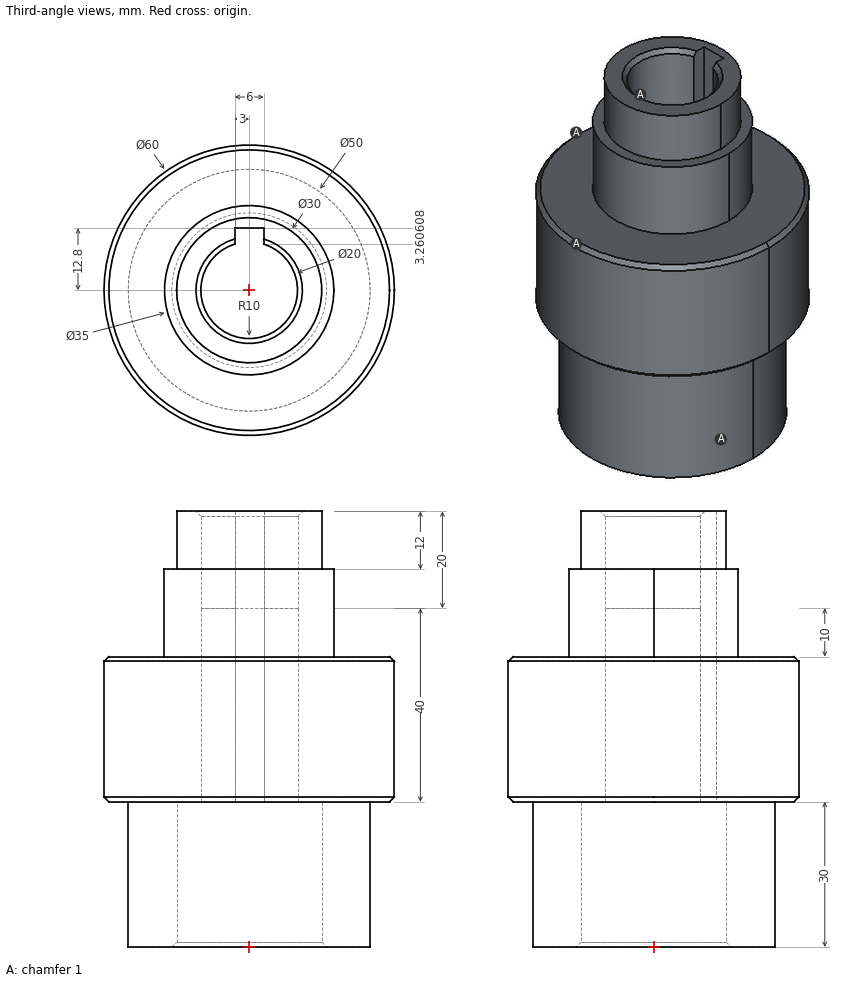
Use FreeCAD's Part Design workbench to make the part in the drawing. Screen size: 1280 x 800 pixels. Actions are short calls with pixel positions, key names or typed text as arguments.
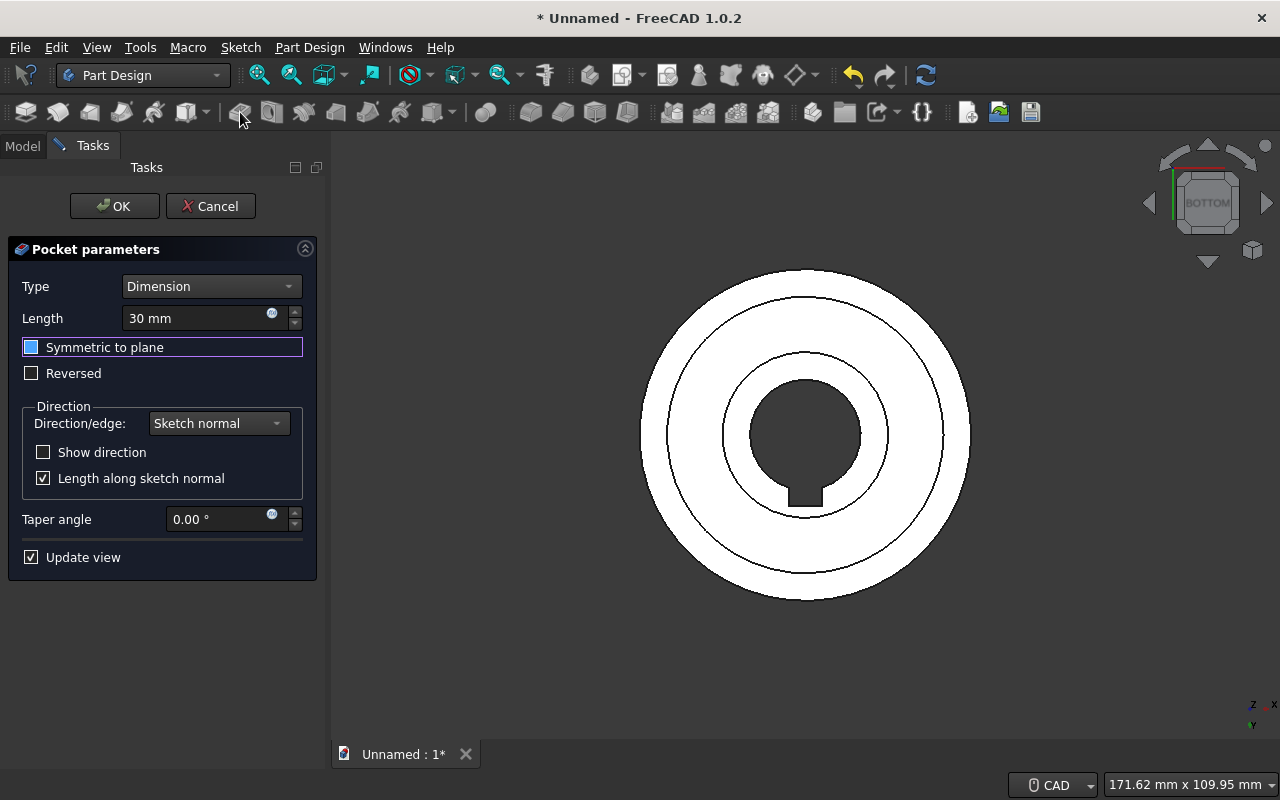
click(115, 206)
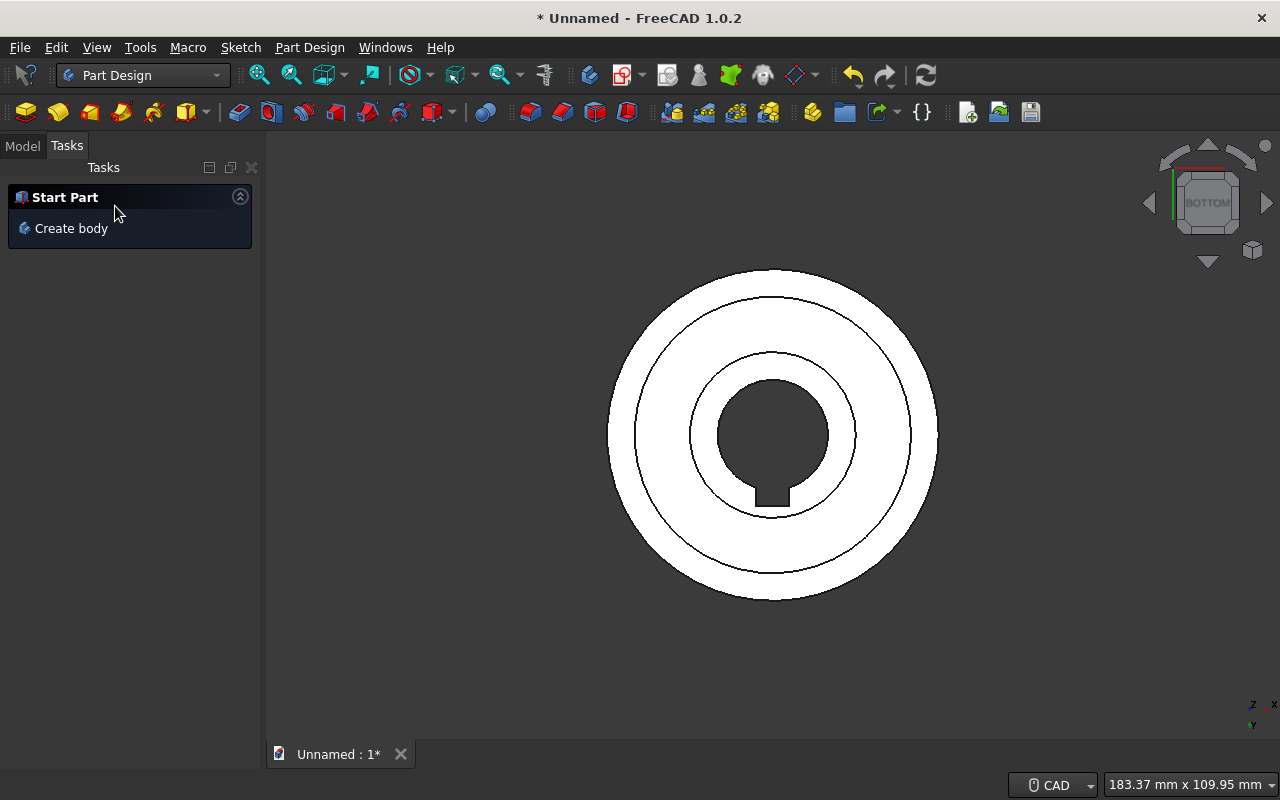
key(0)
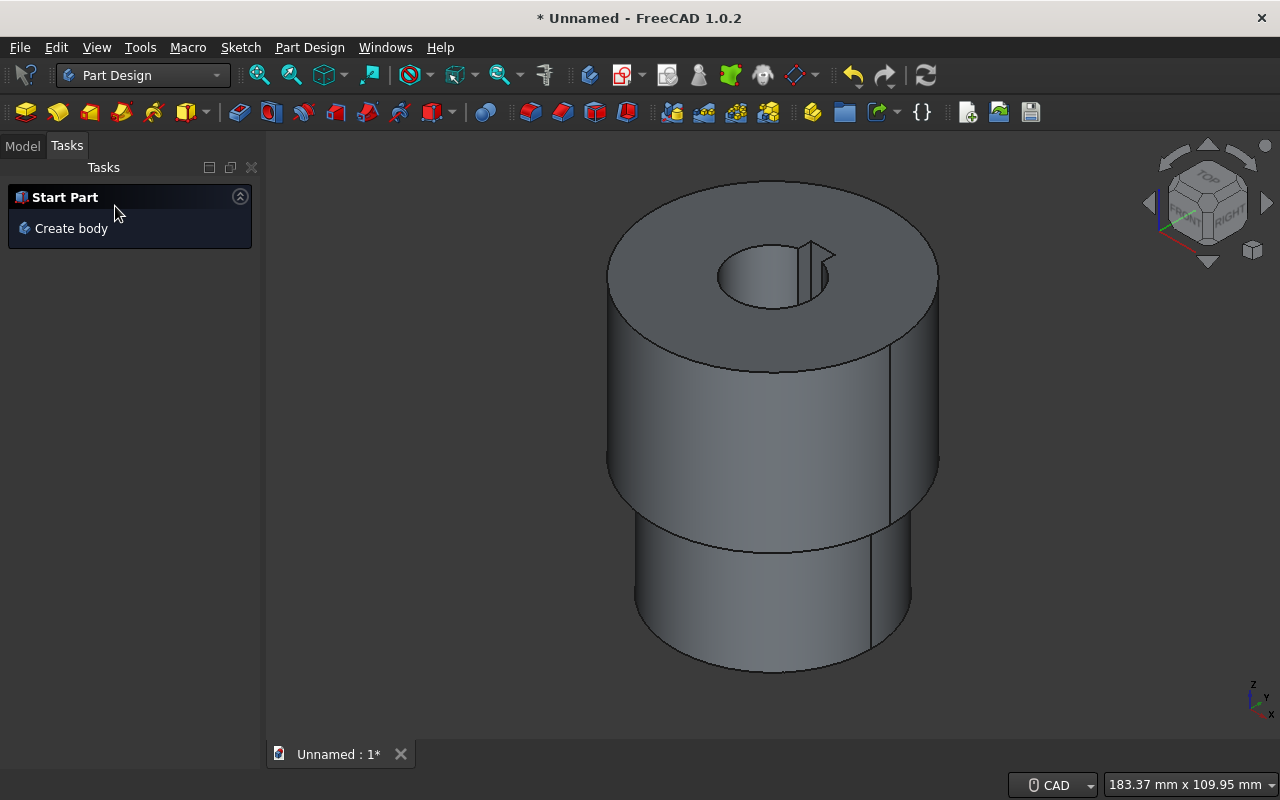
click(806, 334)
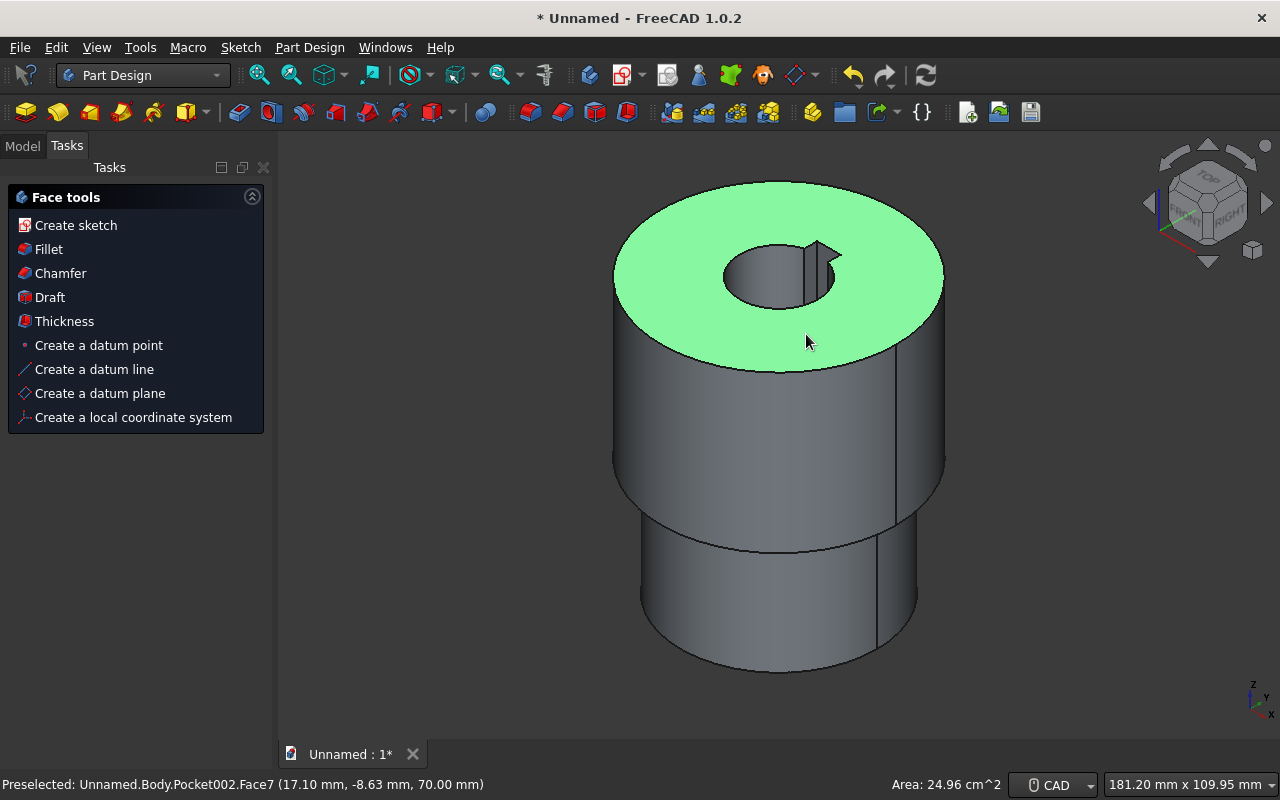
click(622, 76)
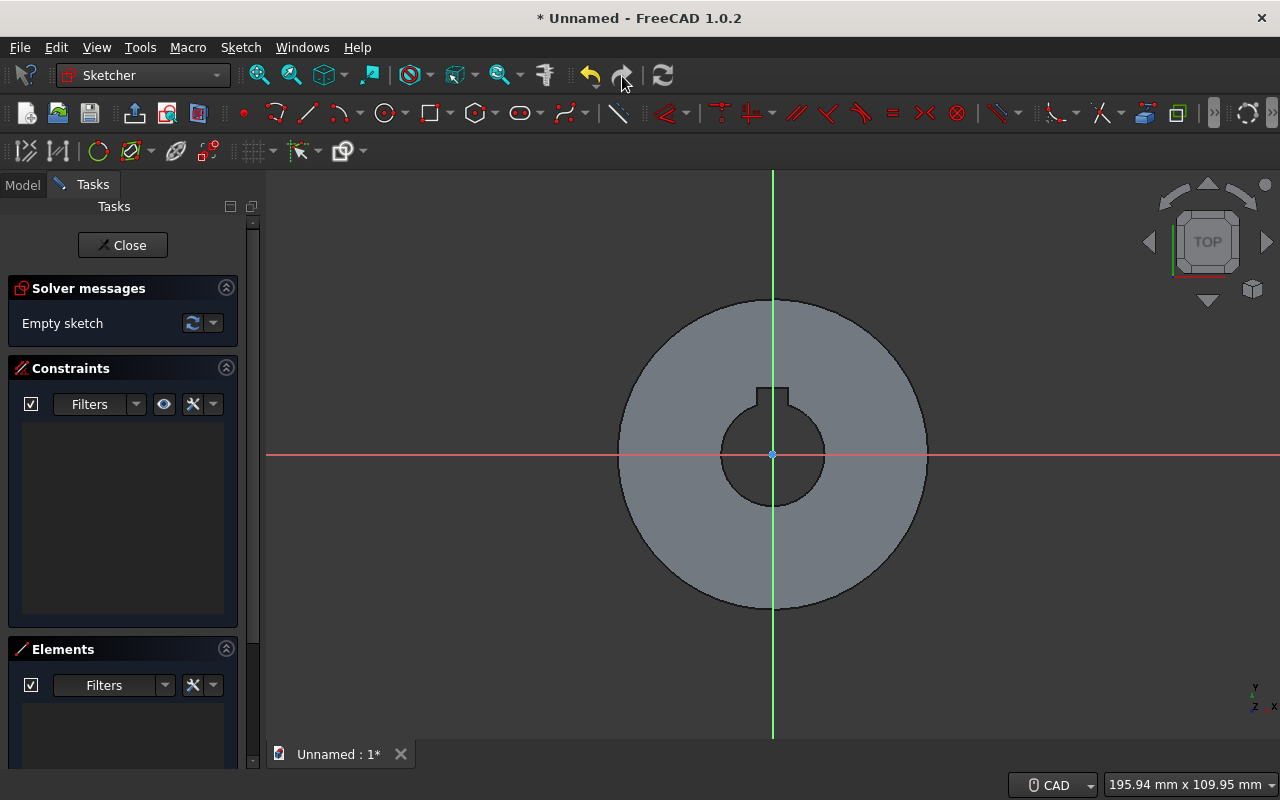
scroll(856, 454, up, 3)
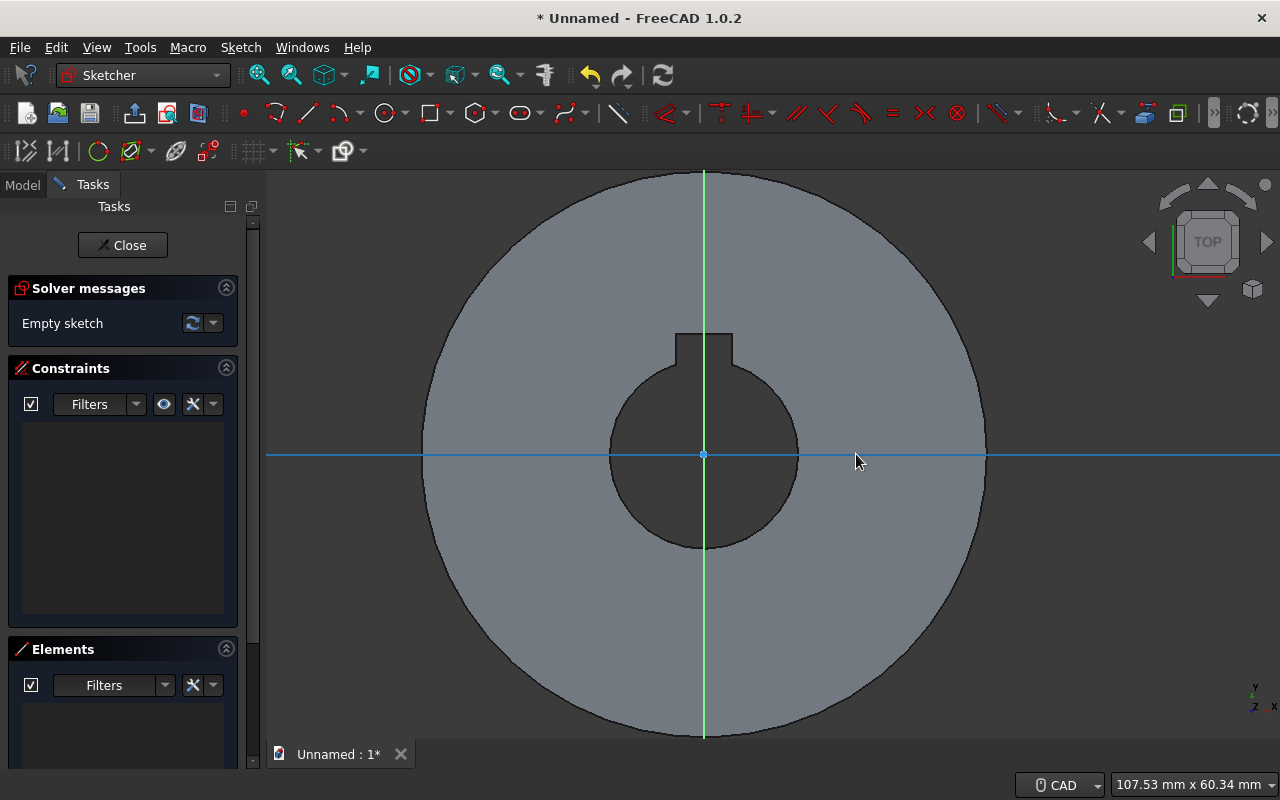
key(g)
key(m)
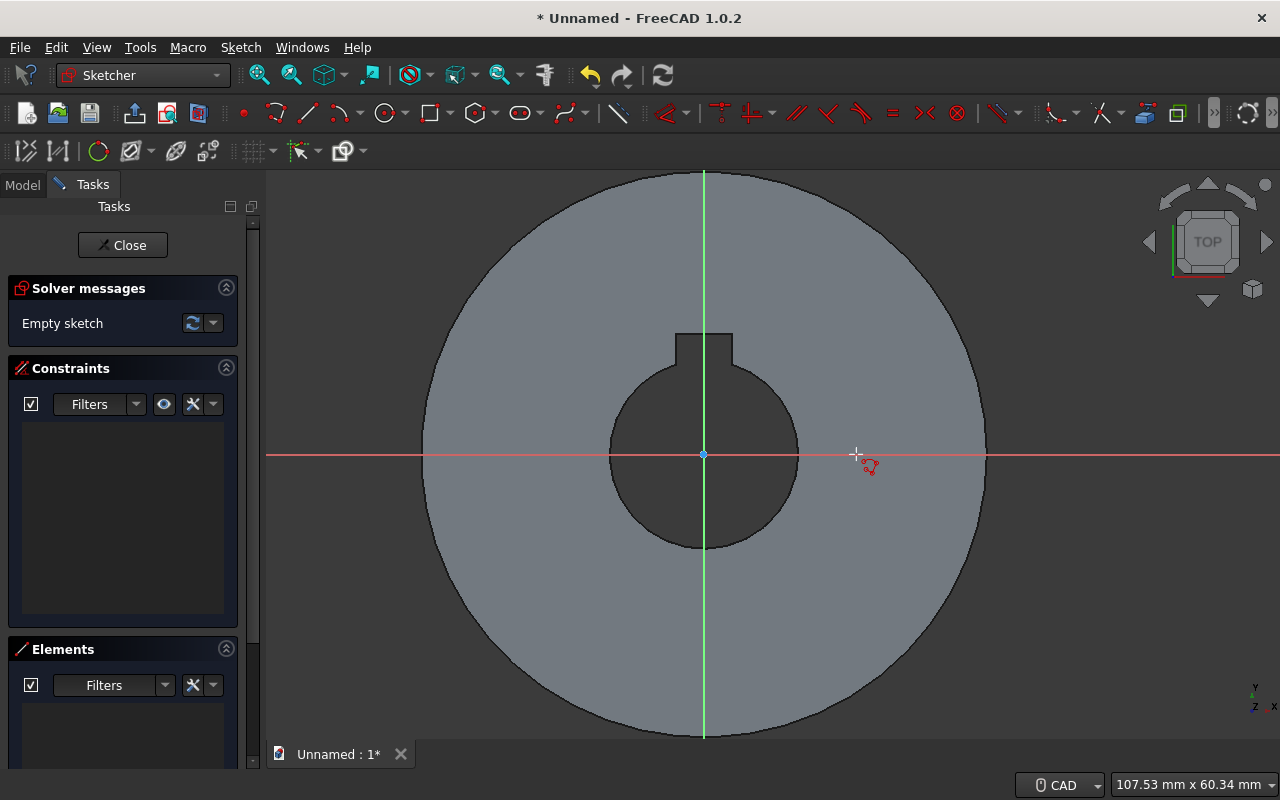
click(676, 365)
click(676, 334)
click(732, 334)
click(732, 365)
right_click(732, 365)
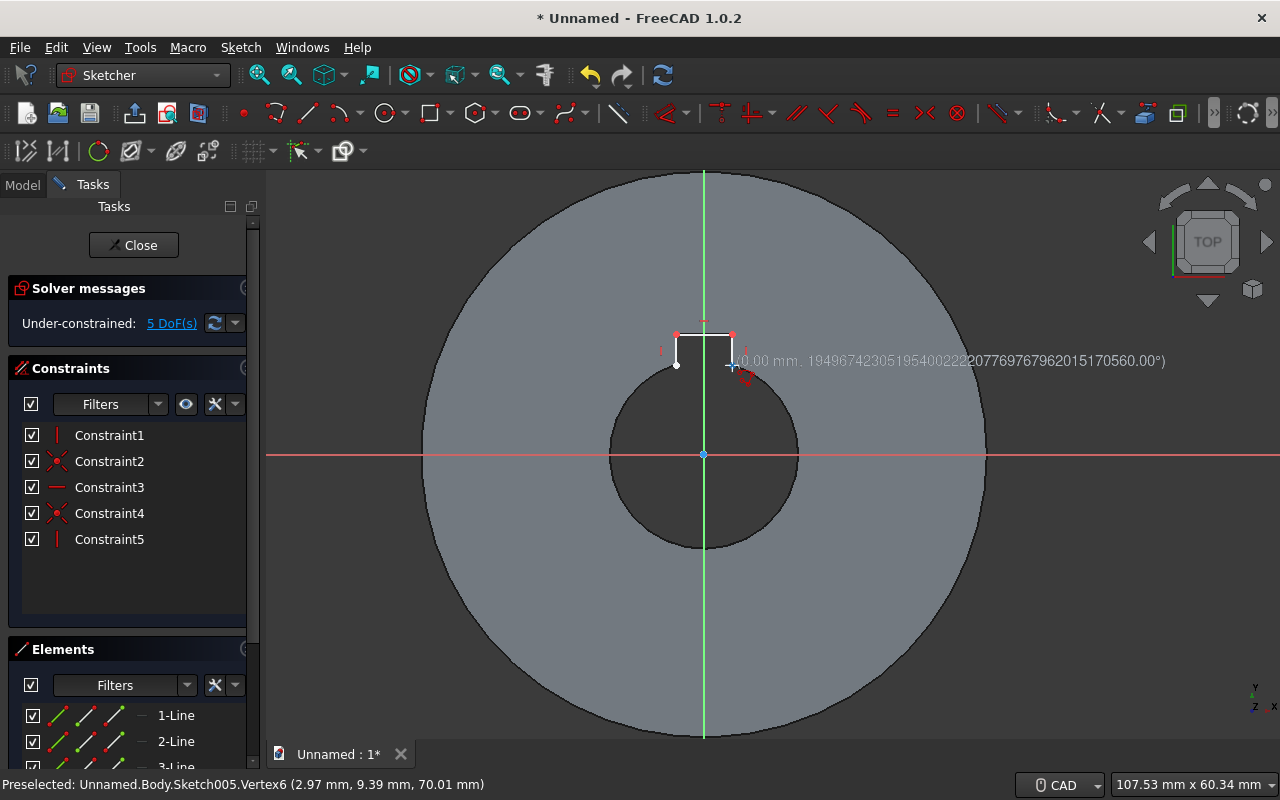
key(g)
key(3)
key(a)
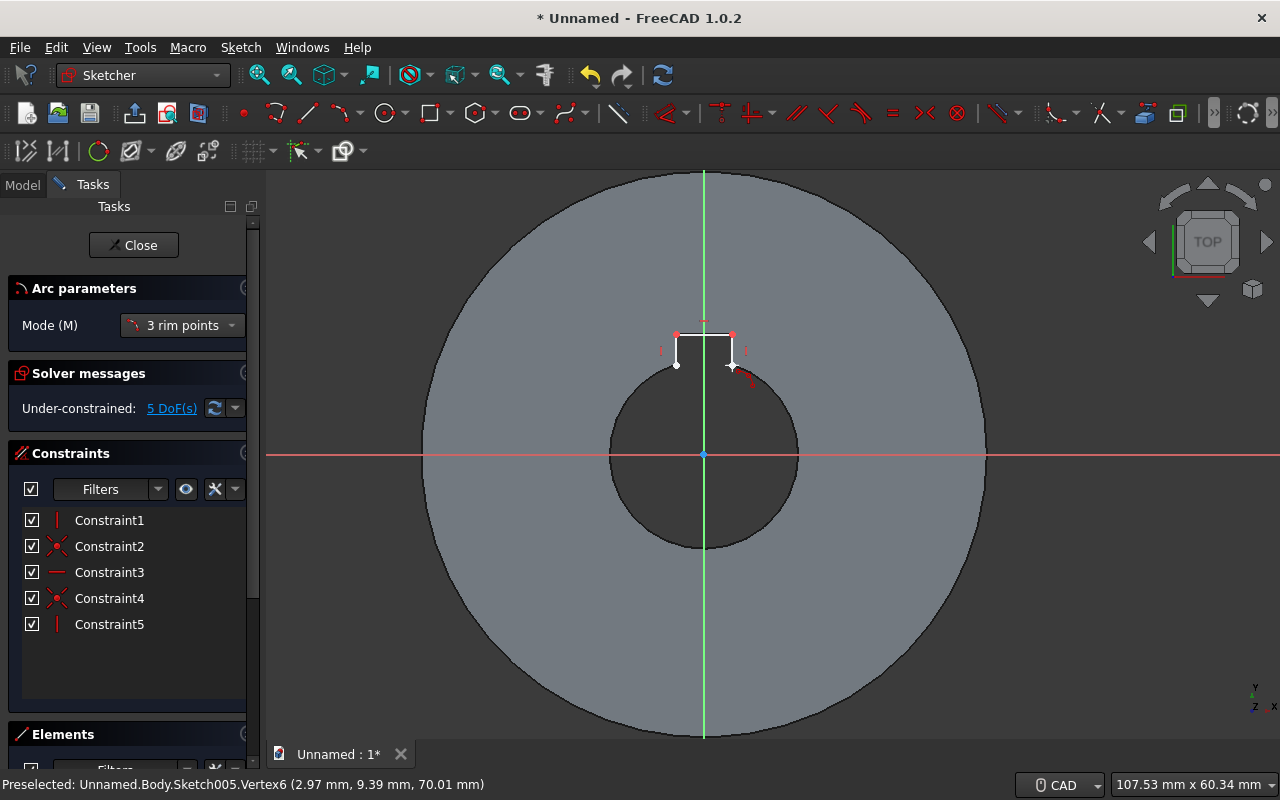
click(732, 366)
click(676, 366)
click(653, 534)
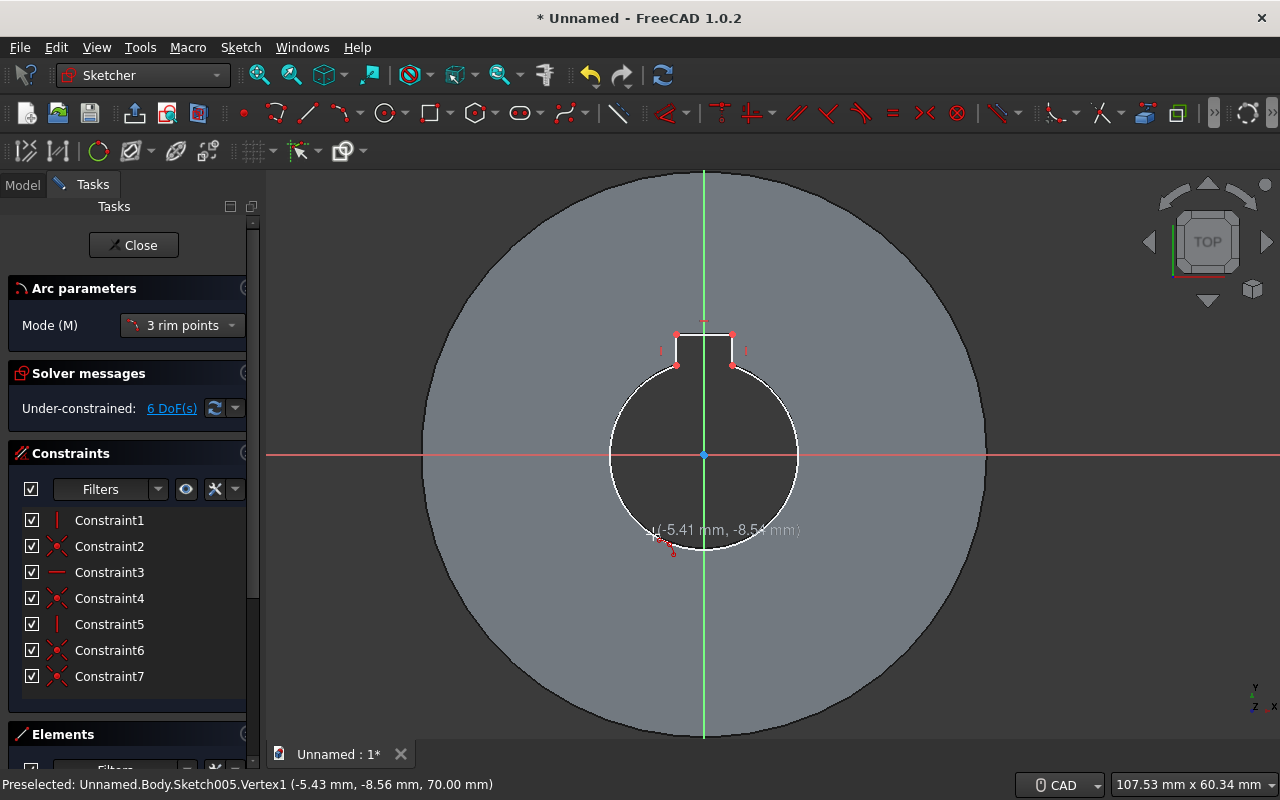
click(386, 114)